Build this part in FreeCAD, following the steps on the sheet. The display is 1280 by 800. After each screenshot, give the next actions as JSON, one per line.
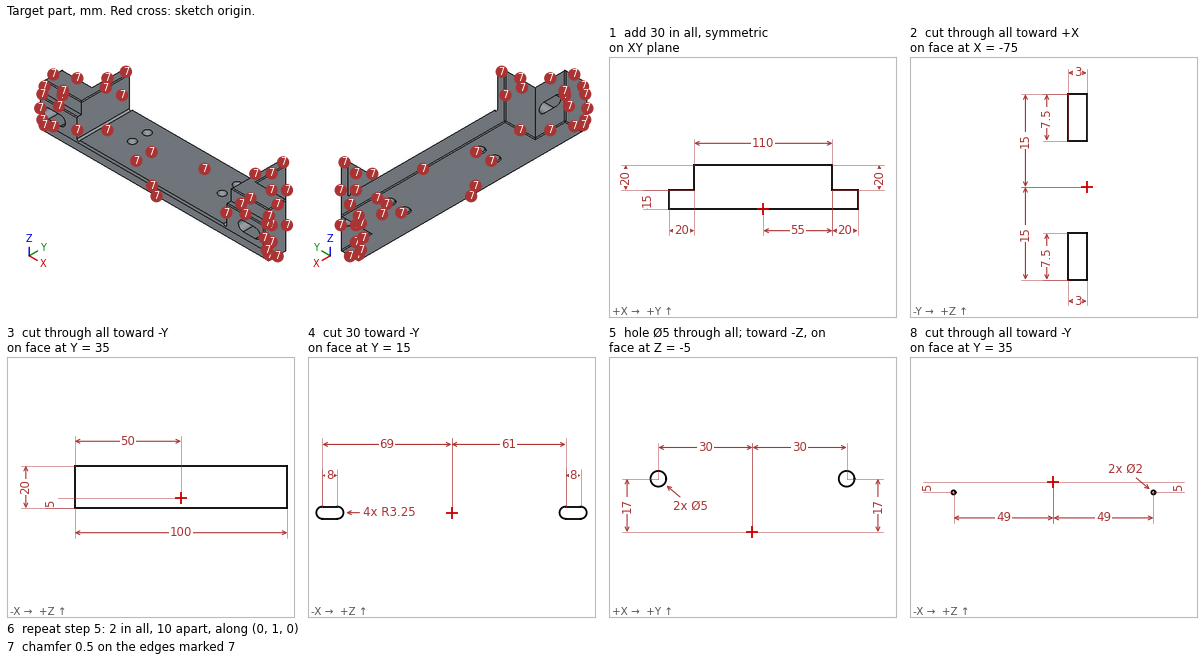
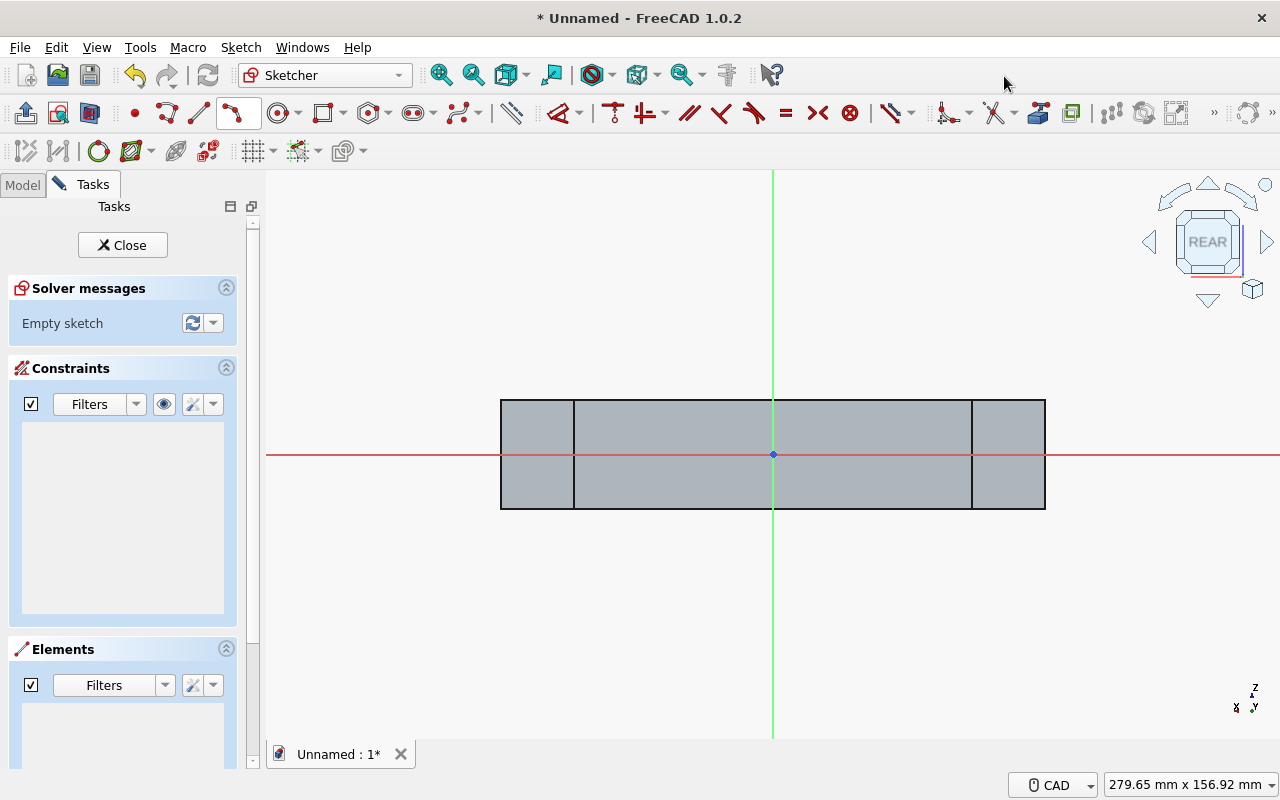
{"action": "scroll", "coordinate": [912, 400], "scroll_direction": "up", "scroll_amount": 2}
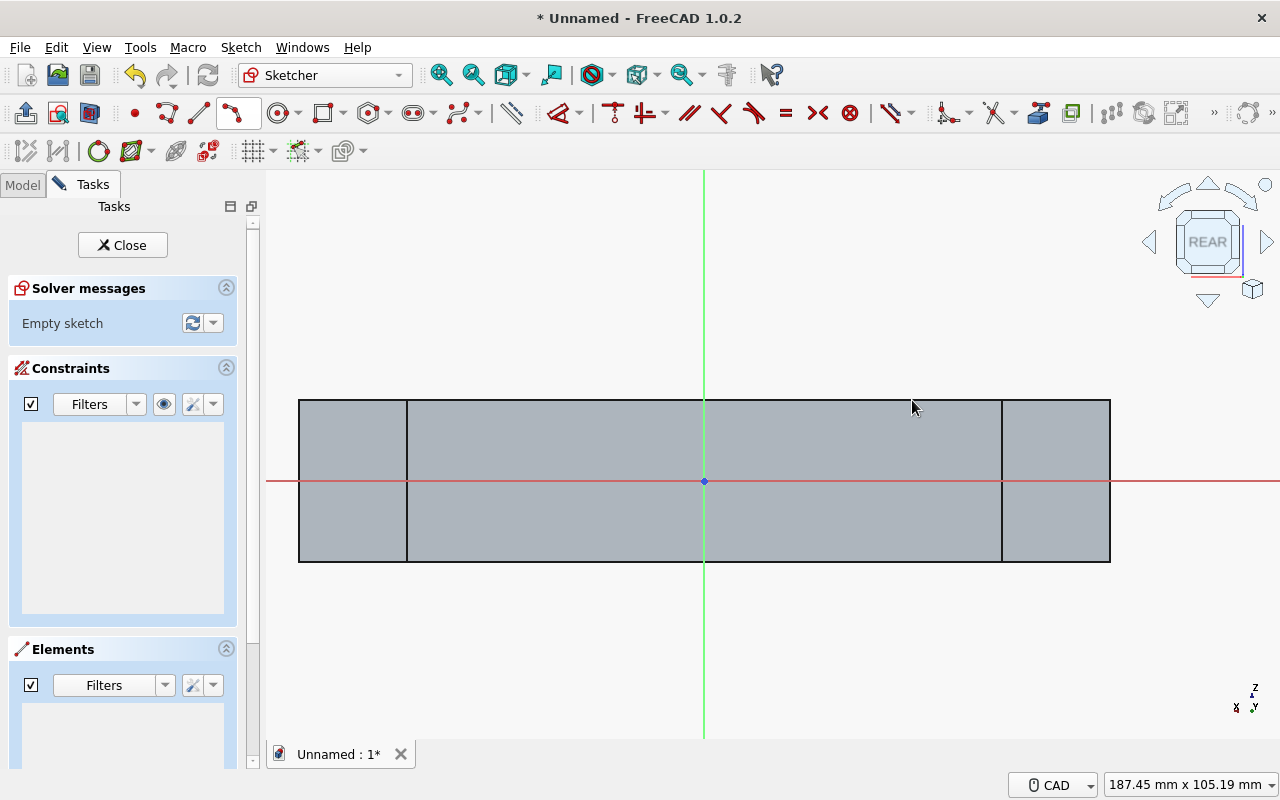
{"action": "key", "text": "g r"}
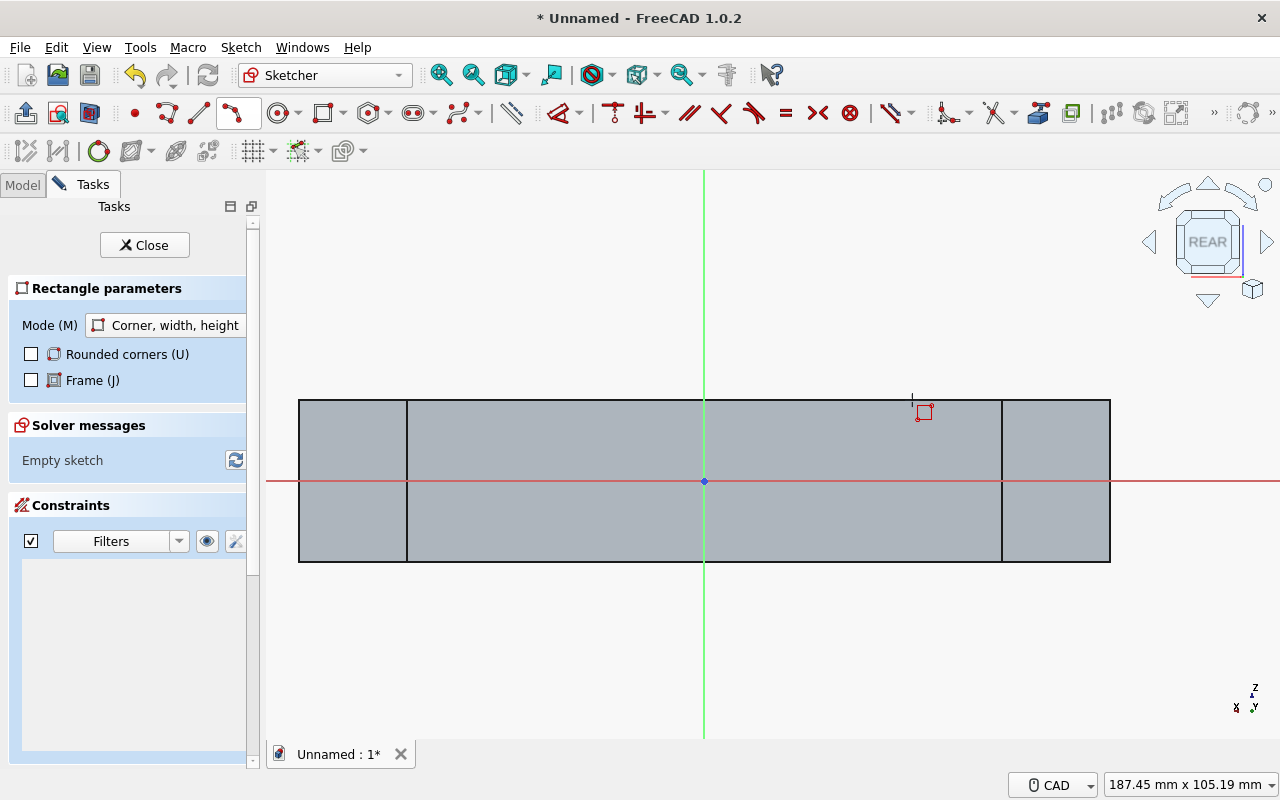
{"action": "left_click", "coordinate": [434, 400]}
{"action": "left_click", "coordinate": [975, 508]}
{"action": "key", "text": "Escape"}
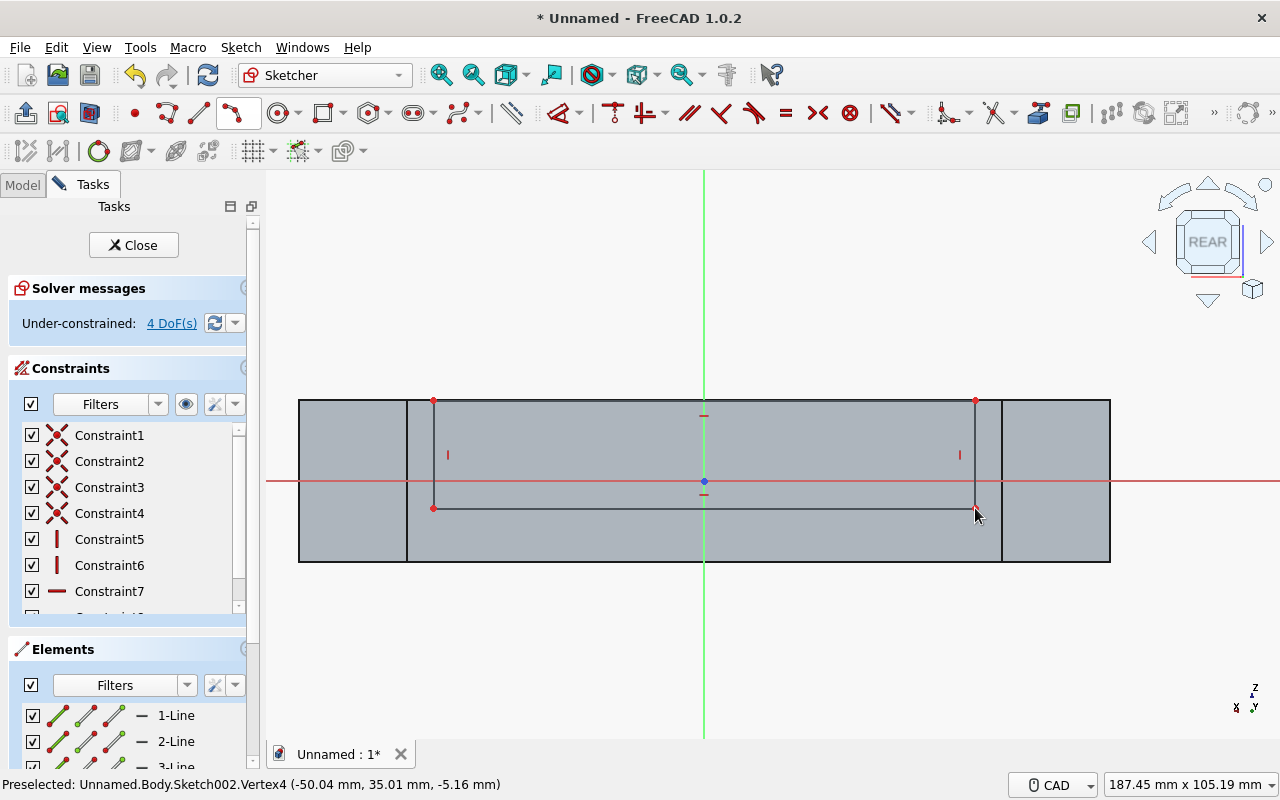
{"action": "left_click", "coordinate": [558, 114]}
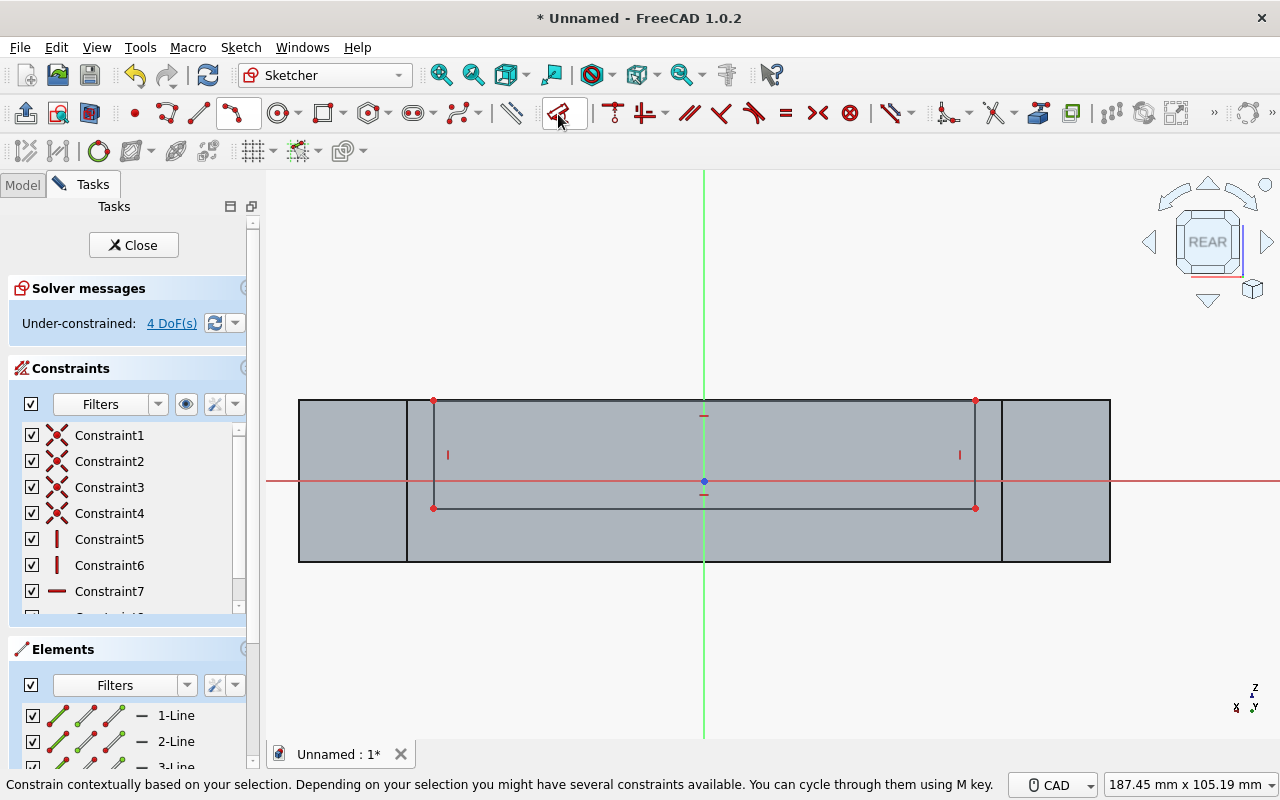
{"action": "left_click", "coordinate": [434, 433]}
{"action": "left_click", "coordinate": [400, 455]}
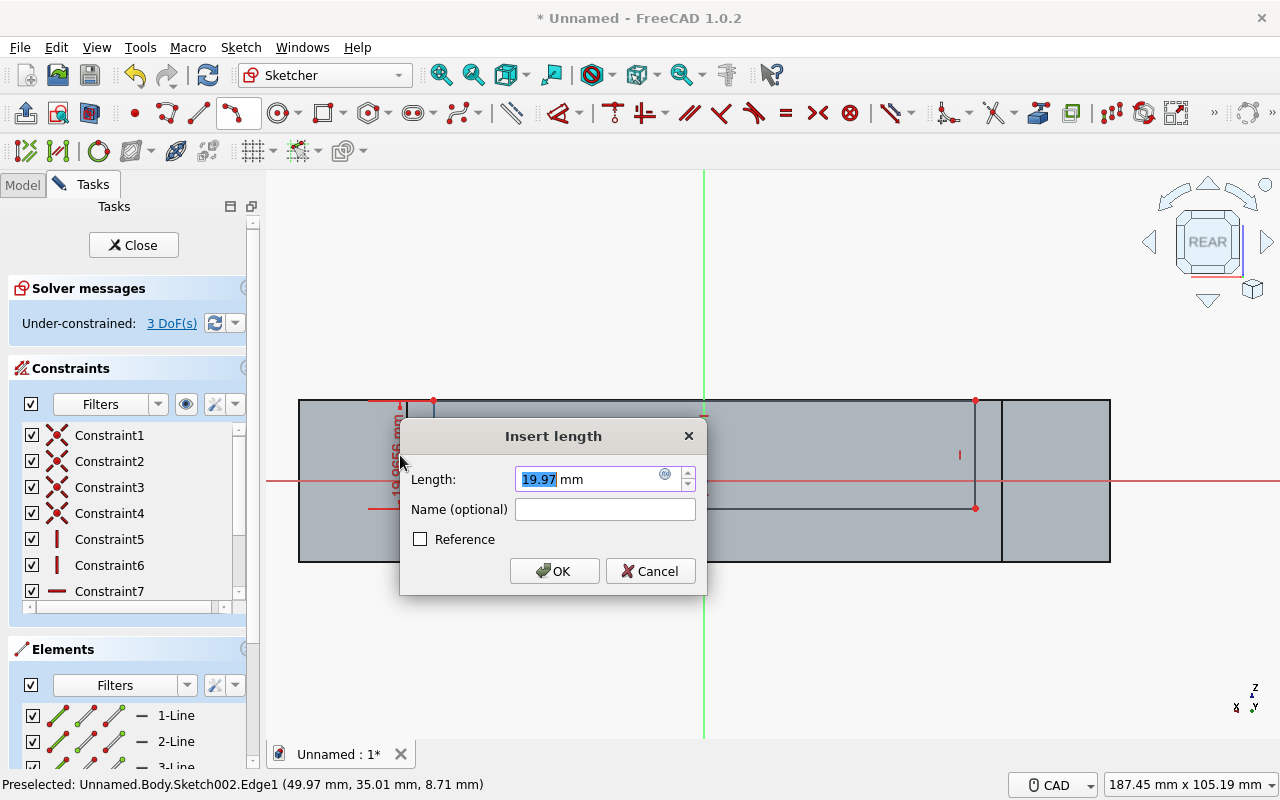
{"action": "type", "text": "20"}
{"action": "key", "text": "Return"}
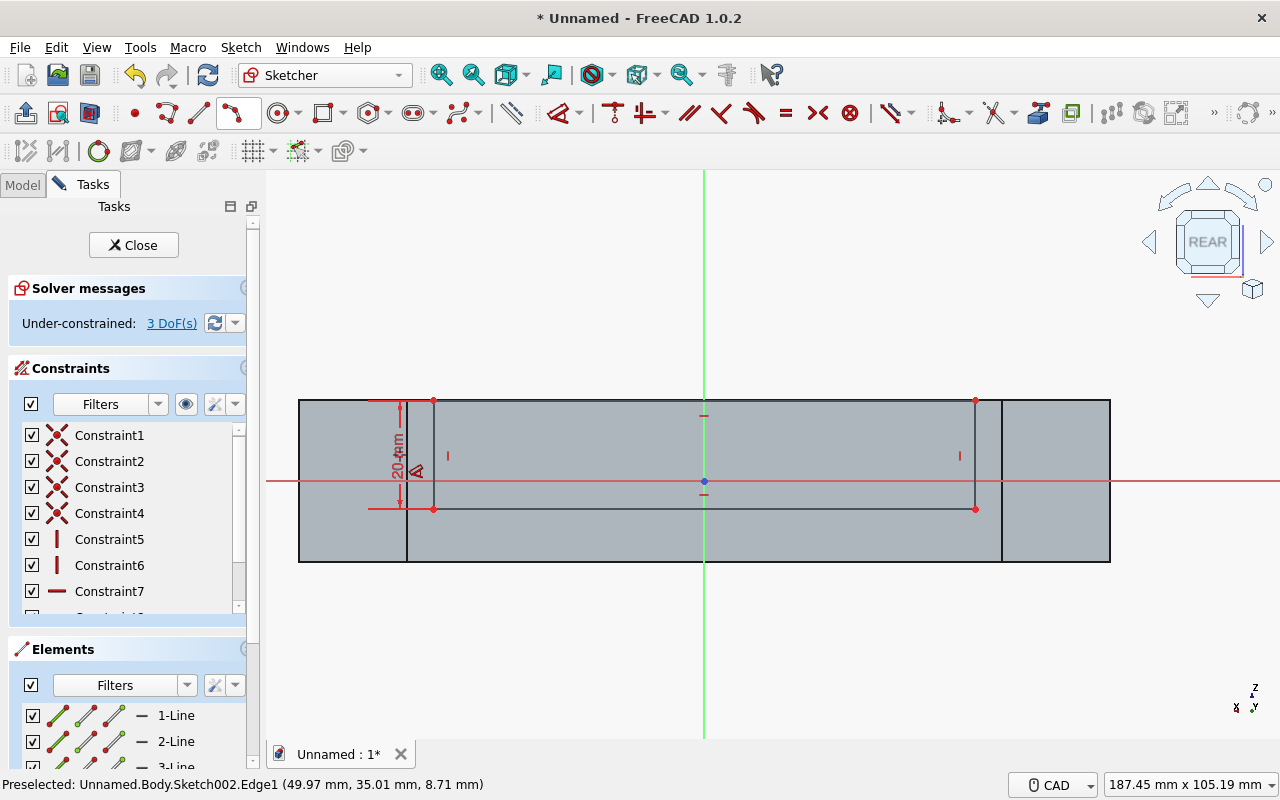
{"action": "scroll", "coordinate": [434, 509], "scroll_direction": "up", "scroll_amount": 2}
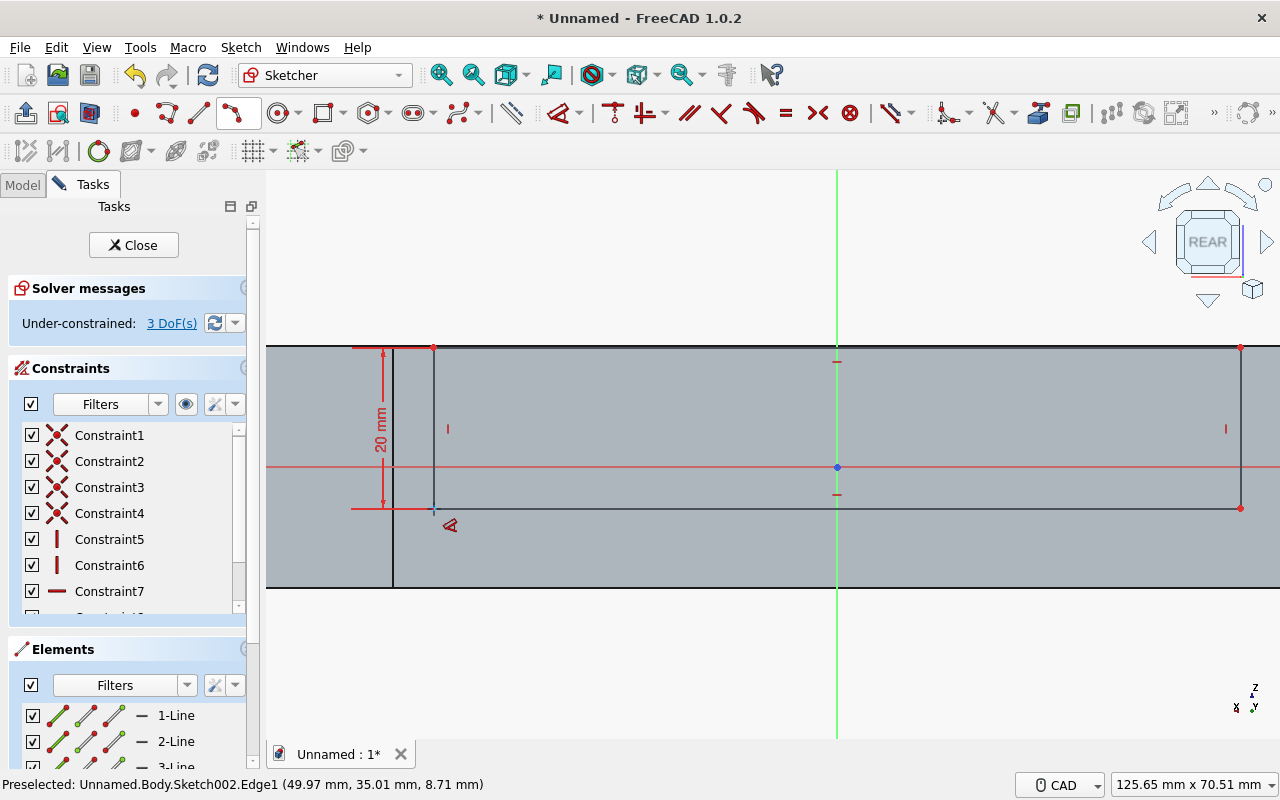
{"action": "left_click", "coordinate": [434, 509]}
{"action": "left_click", "coordinate": [400, 488]}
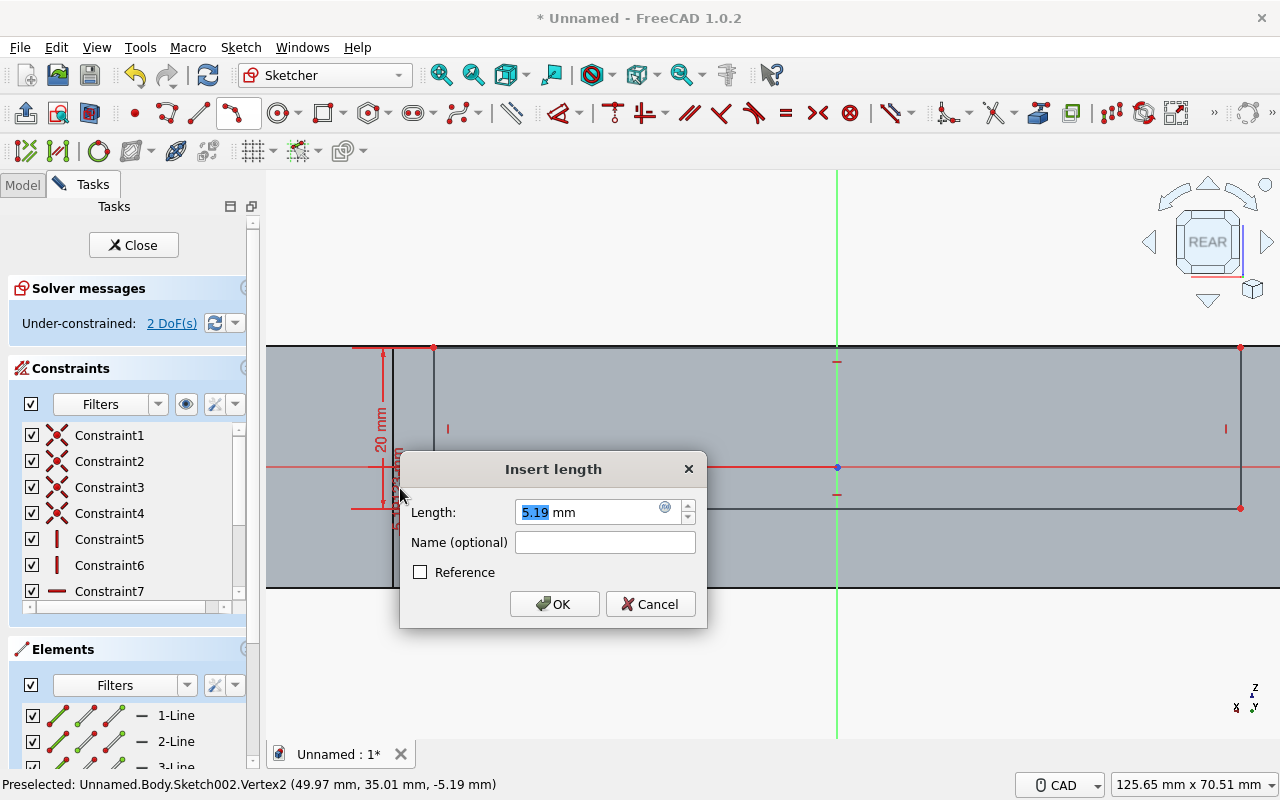
{"action": "type", "text": "5"}
{"action": "key", "text": "Return"}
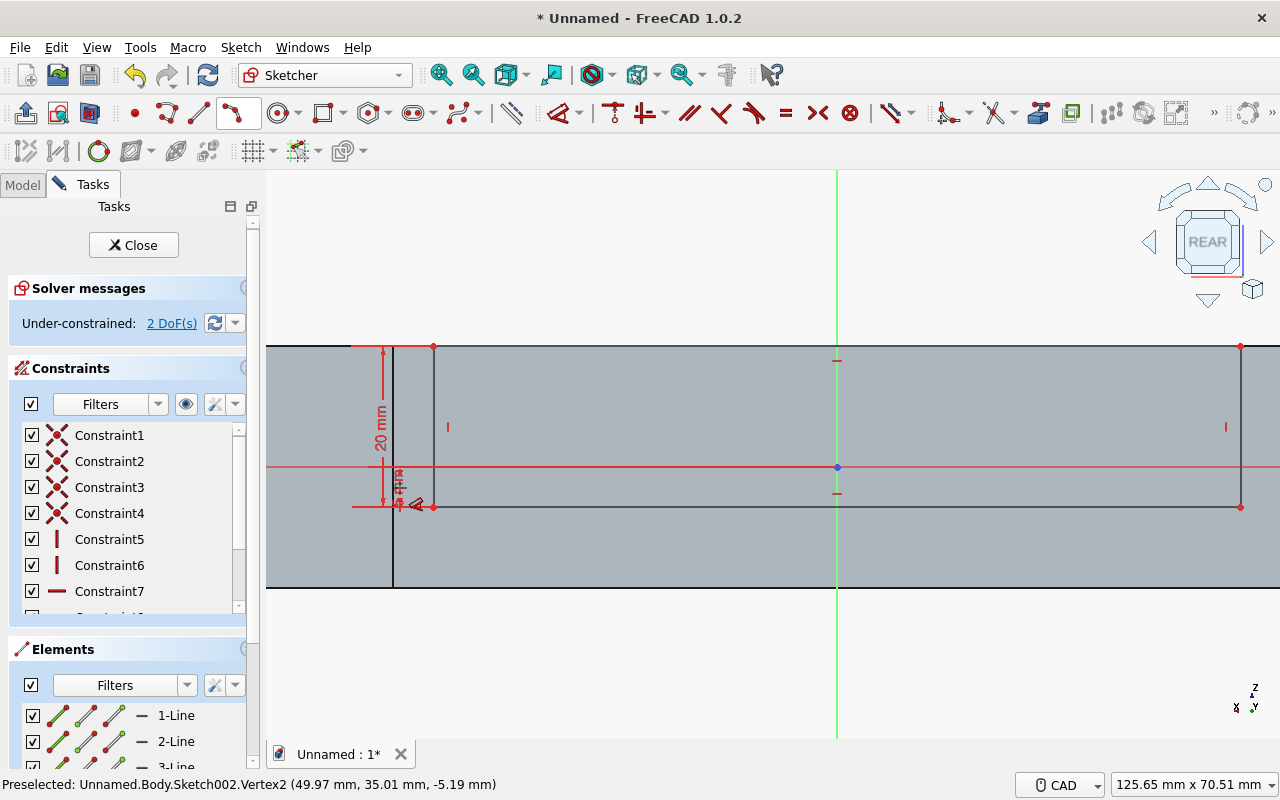
{"action": "left_click", "coordinate": [676, 507]}
{"action": "left_click", "coordinate": [774, 541]}